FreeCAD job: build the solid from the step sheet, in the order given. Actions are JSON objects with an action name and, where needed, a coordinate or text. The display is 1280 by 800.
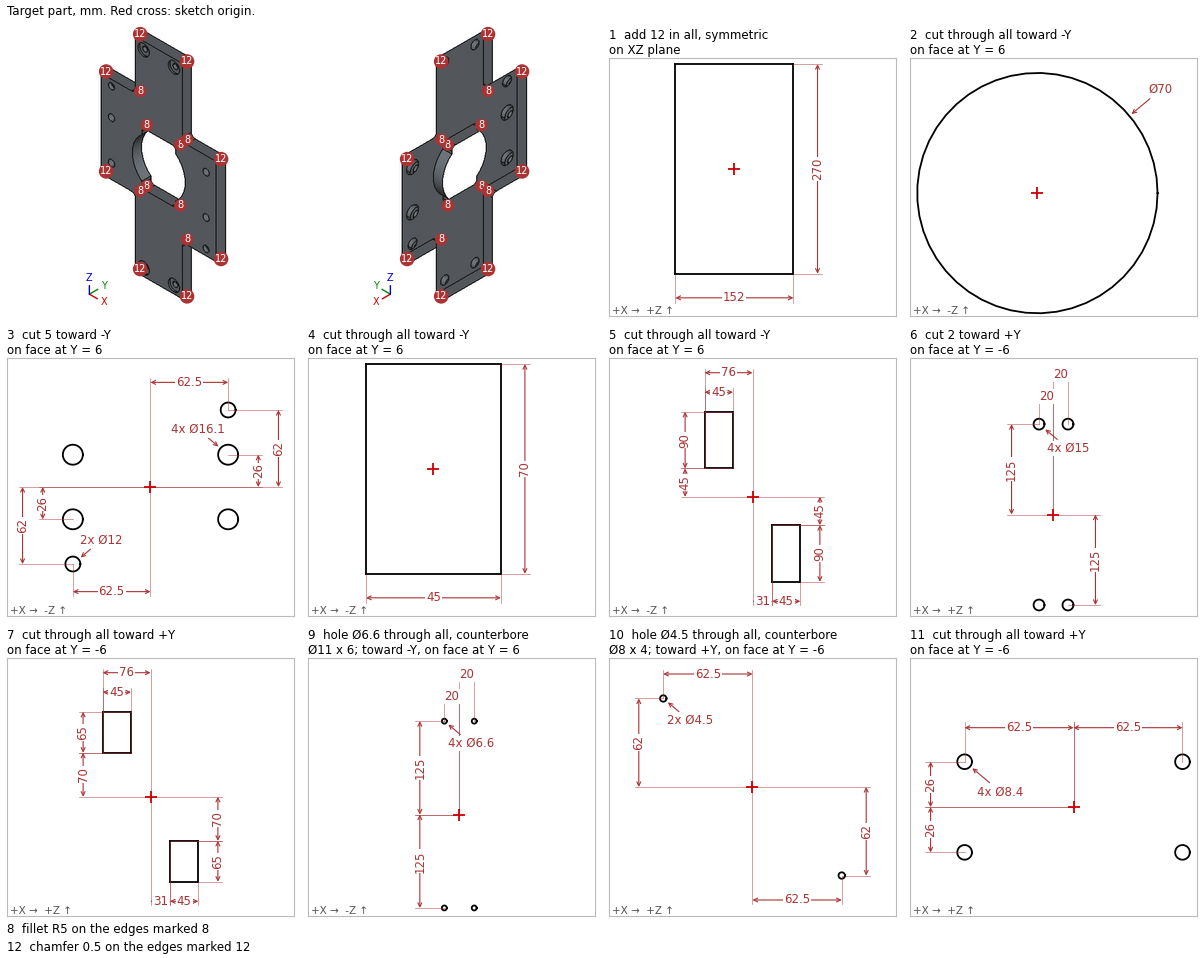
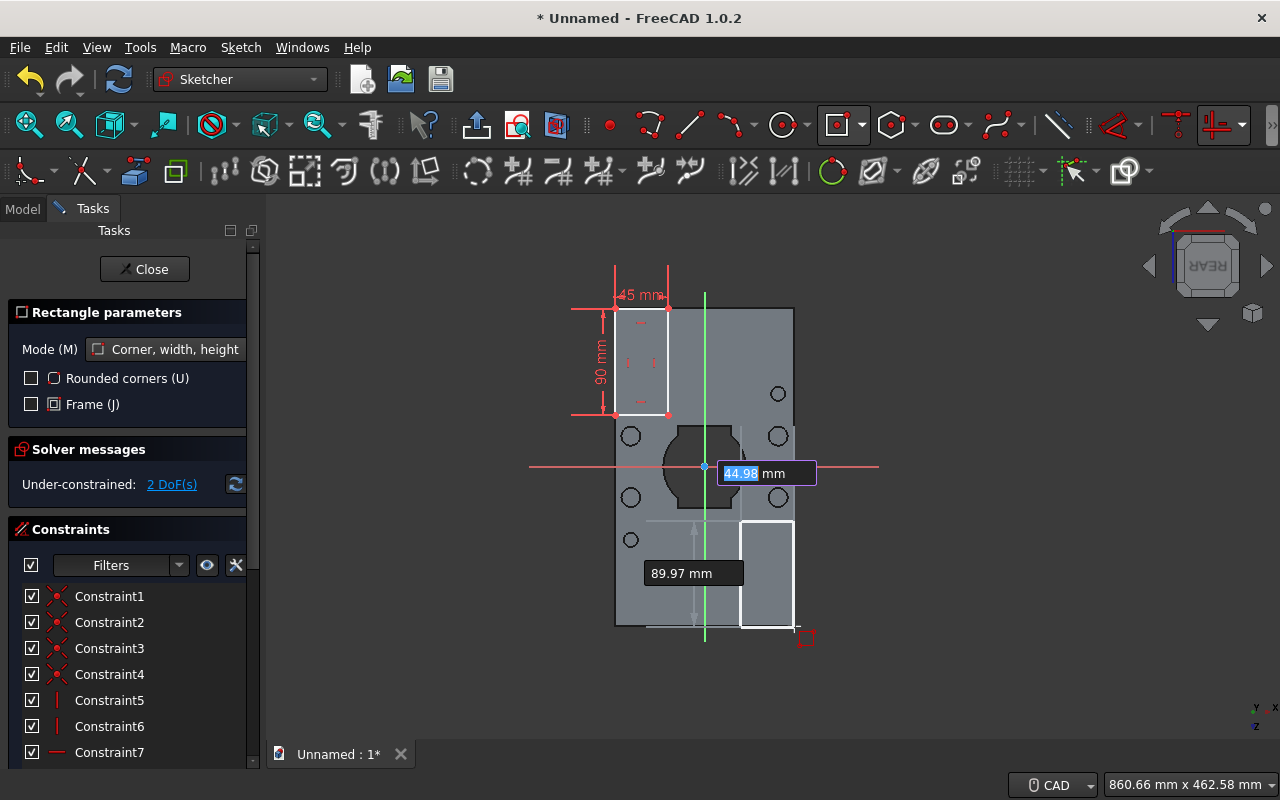
{"action": "type", "text": "45"}
{"action": "key", "text": "Tab"}
{"action": "type", "text": "90"}
{"action": "key", "text": "Return"}
{"action": "key", "text": "Escape"}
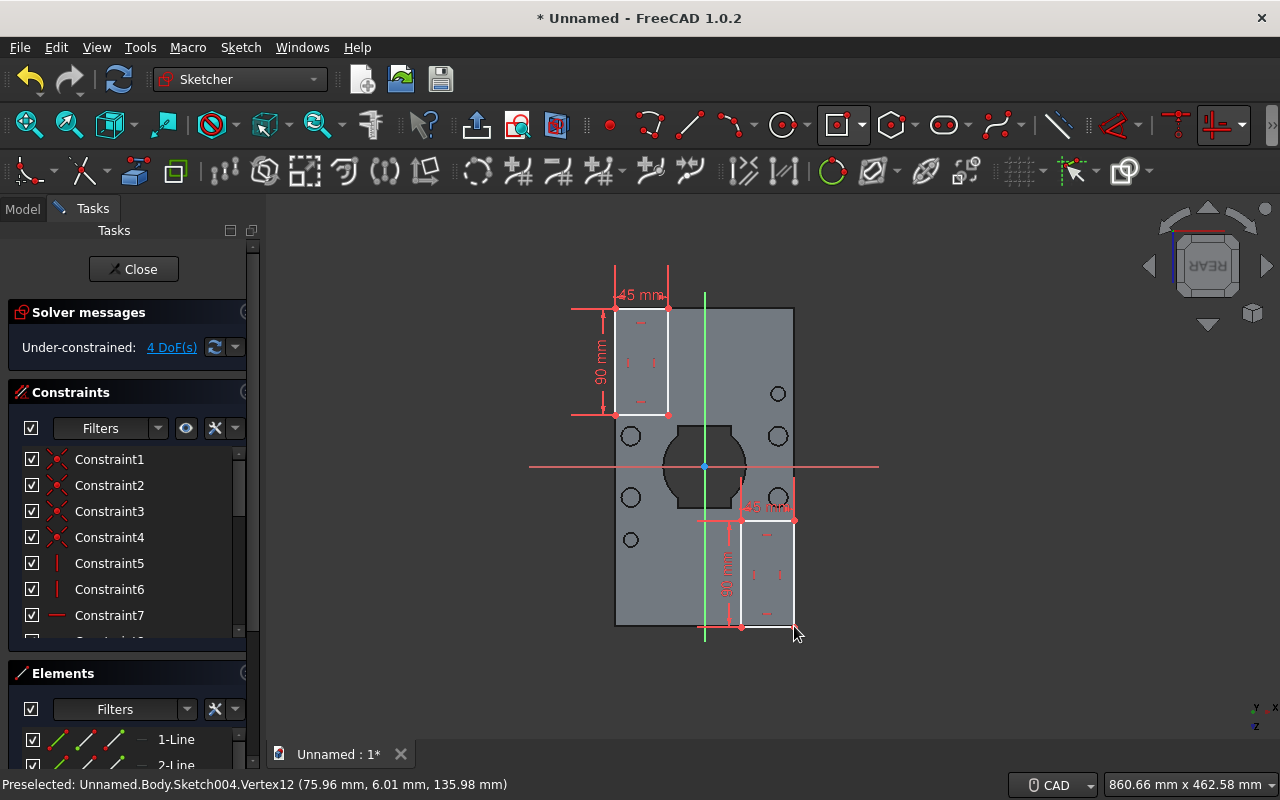
{"action": "key", "text": "d"}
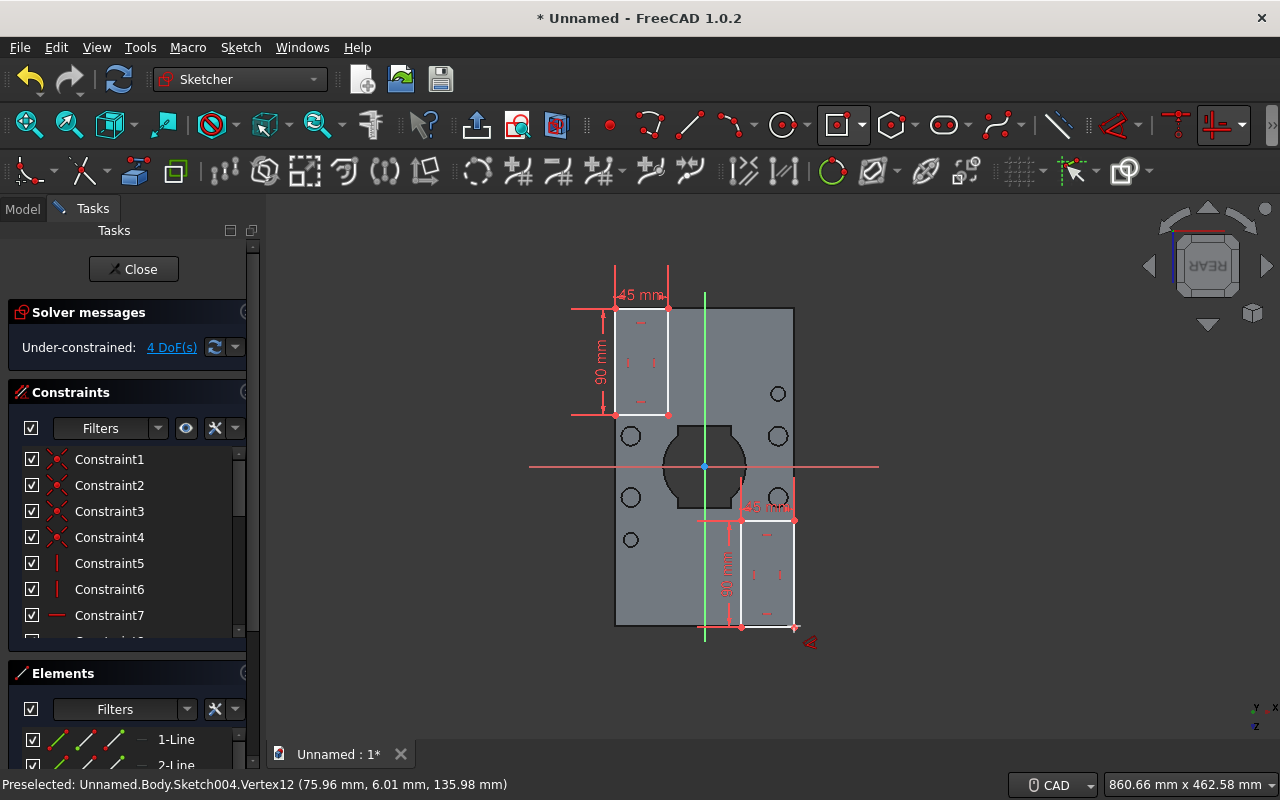
{"action": "left_click", "coordinate": [615, 309]}
{"action": "left_click", "coordinate": [660, 275]}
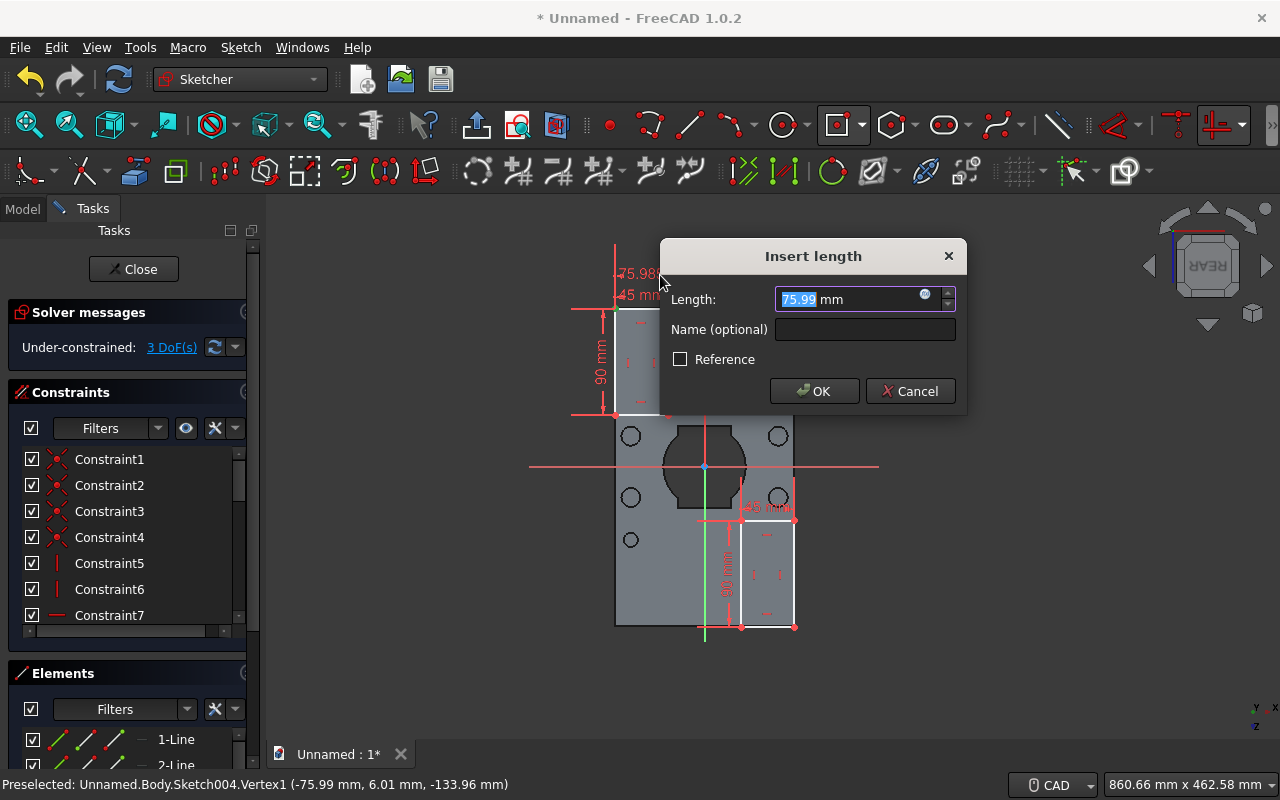
{"action": "type", "text": "76"}
{"action": "key", "text": "Return"}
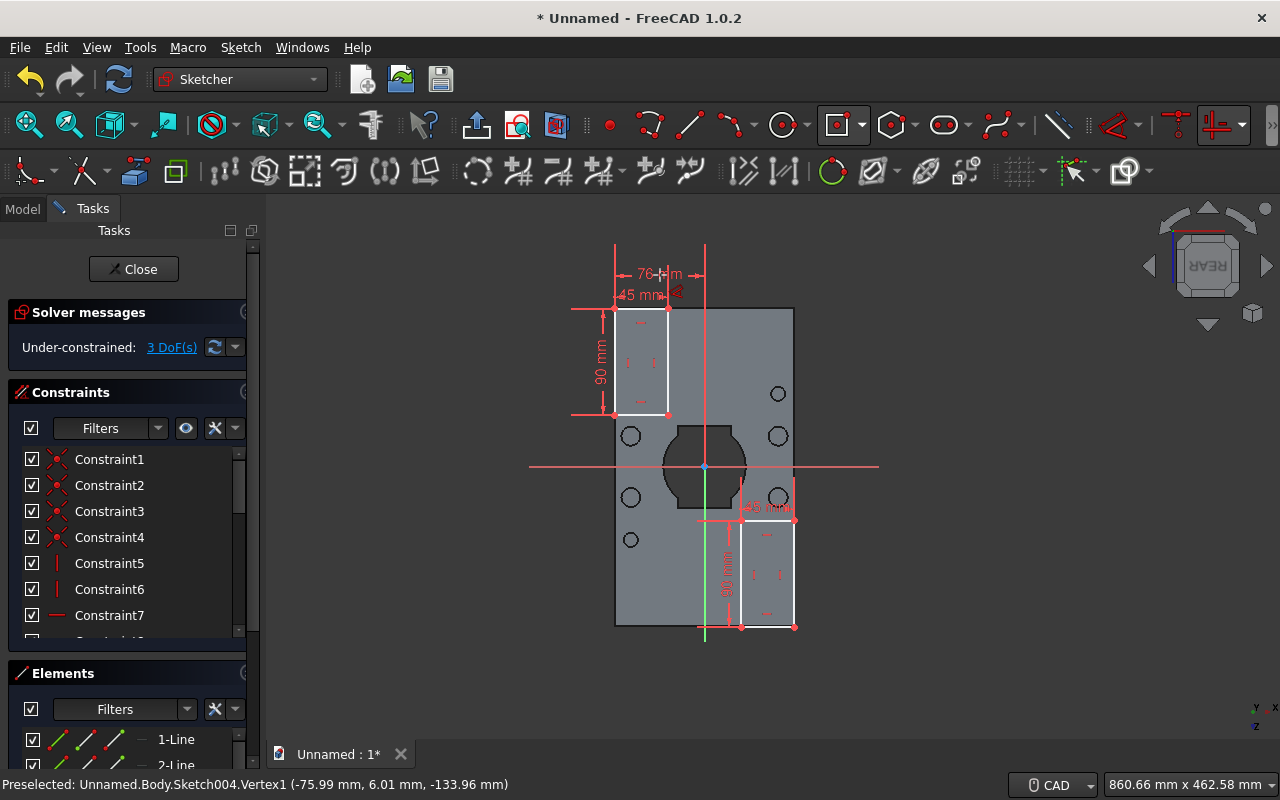
{"action": "left_click", "coordinate": [615, 415]}
{"action": "left_click", "coordinate": [581, 441]}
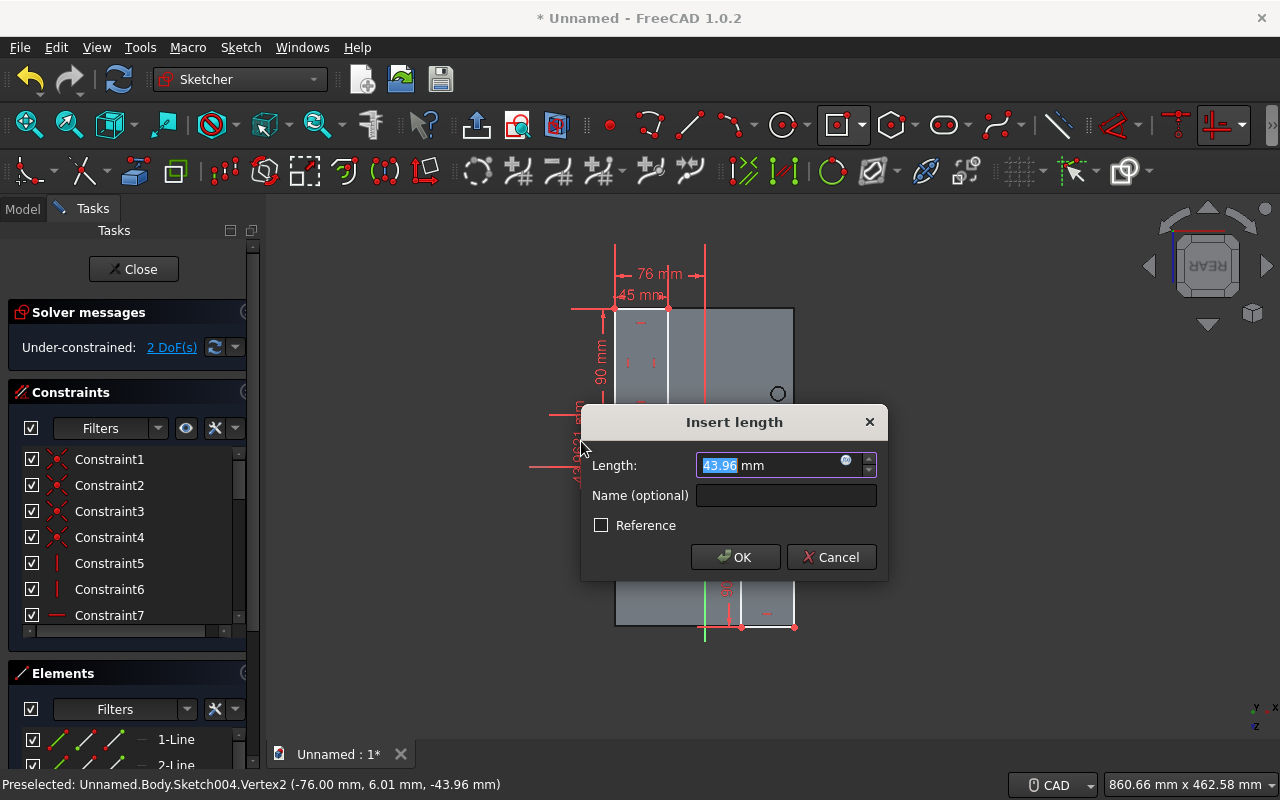
{"action": "type", "text": "45"}
{"action": "key", "text": "Return"}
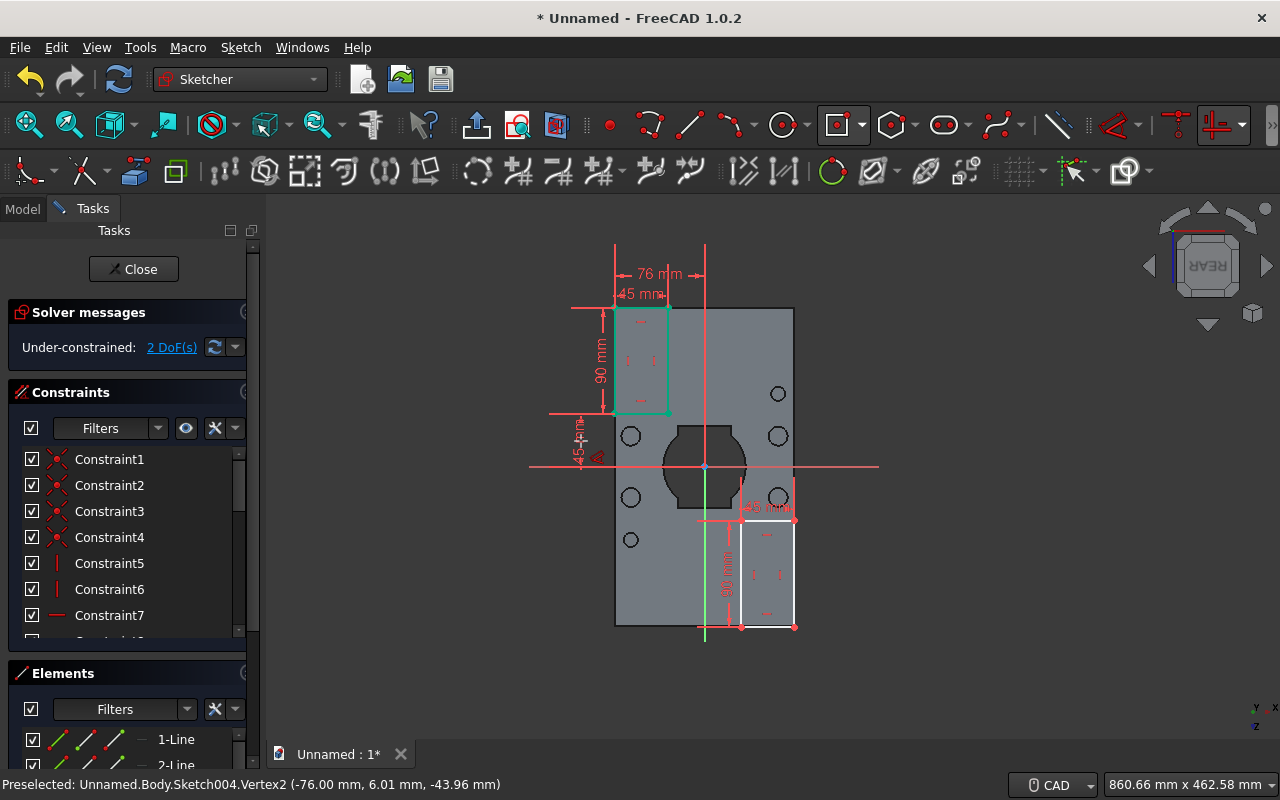
{"action": "left_click", "coordinate": [741, 521]}
{"action": "left_click", "coordinate": [723, 555]}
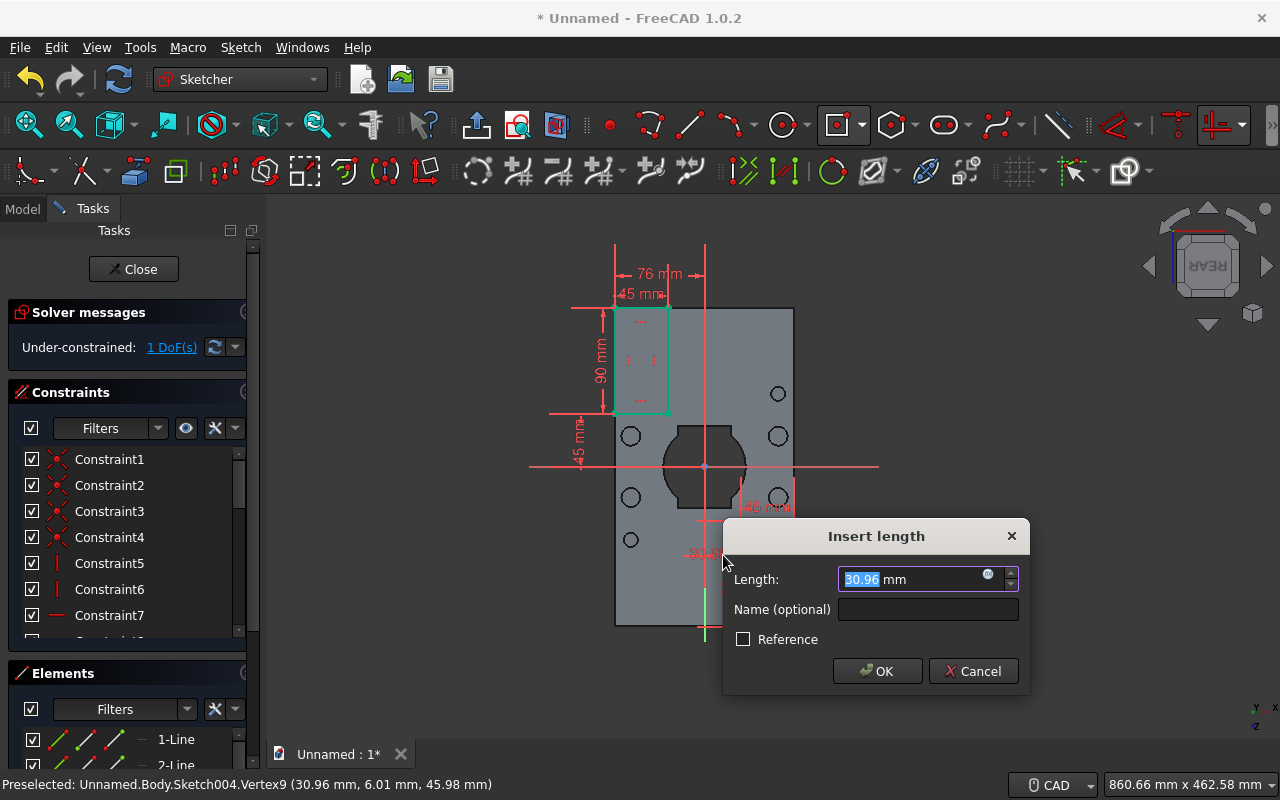
{"action": "type", "text": "31"}
{"action": "key", "text": "Return"}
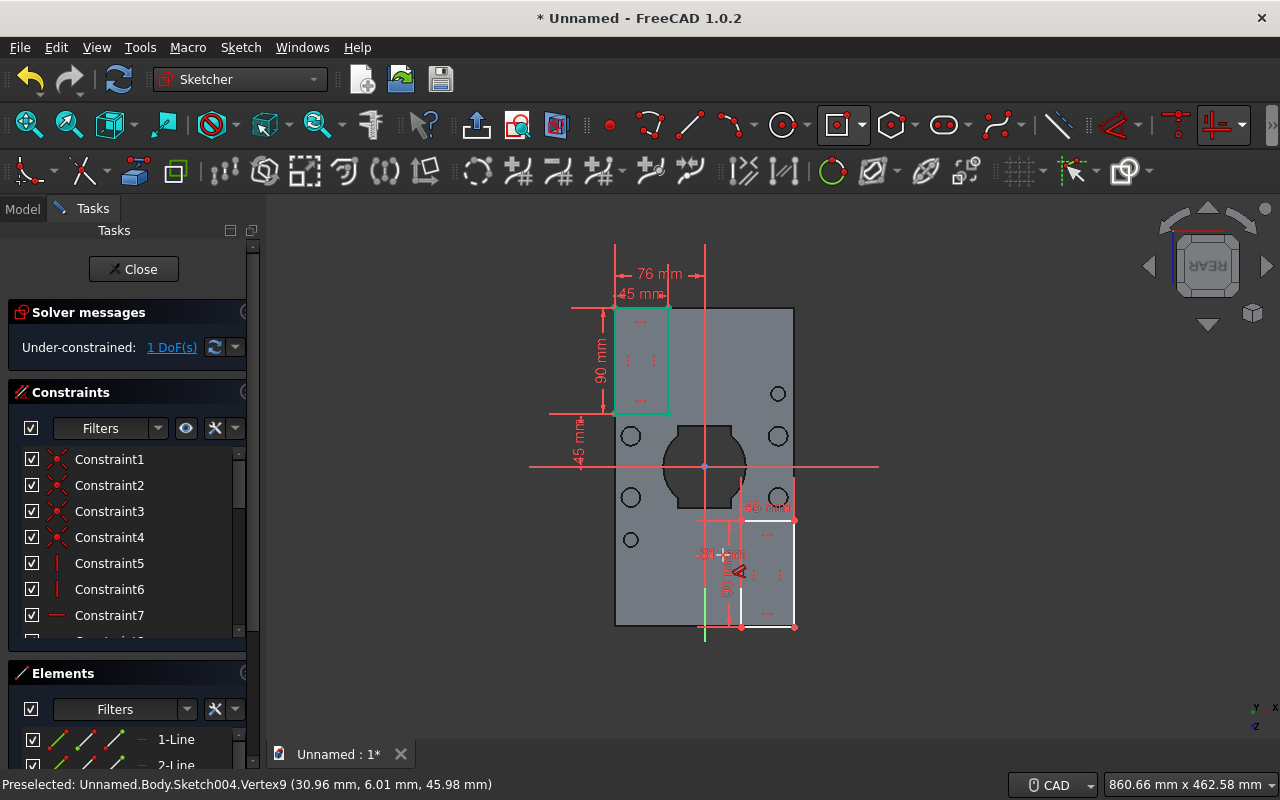
{"action": "left_click", "coordinate": [741, 521]}
{"action": "left_click", "coordinate": [775, 494]}